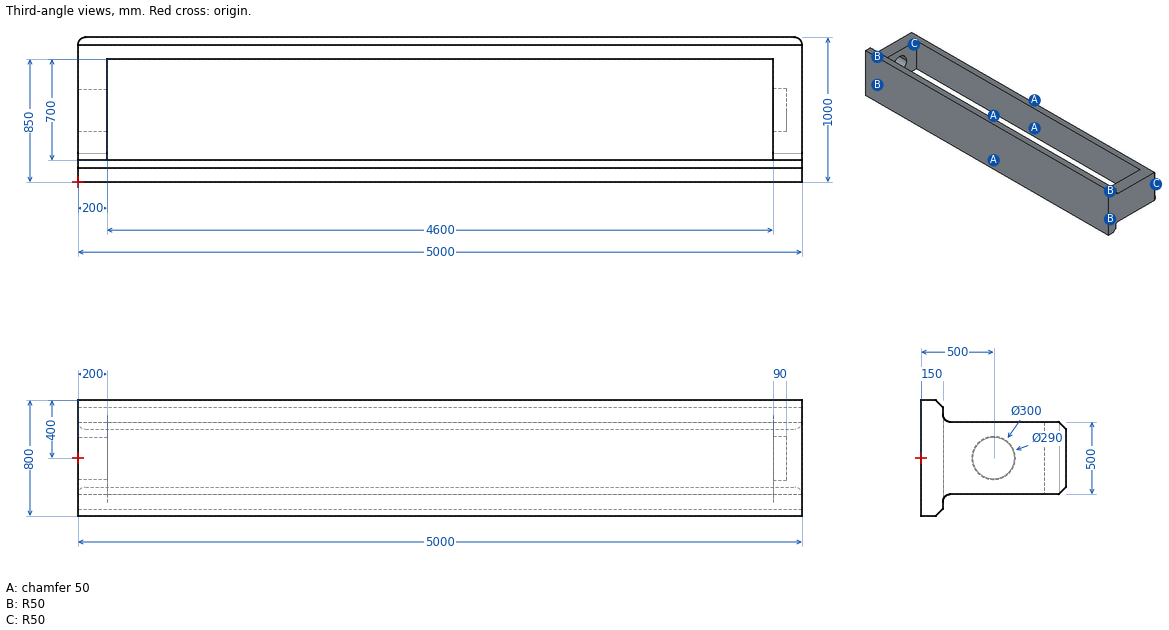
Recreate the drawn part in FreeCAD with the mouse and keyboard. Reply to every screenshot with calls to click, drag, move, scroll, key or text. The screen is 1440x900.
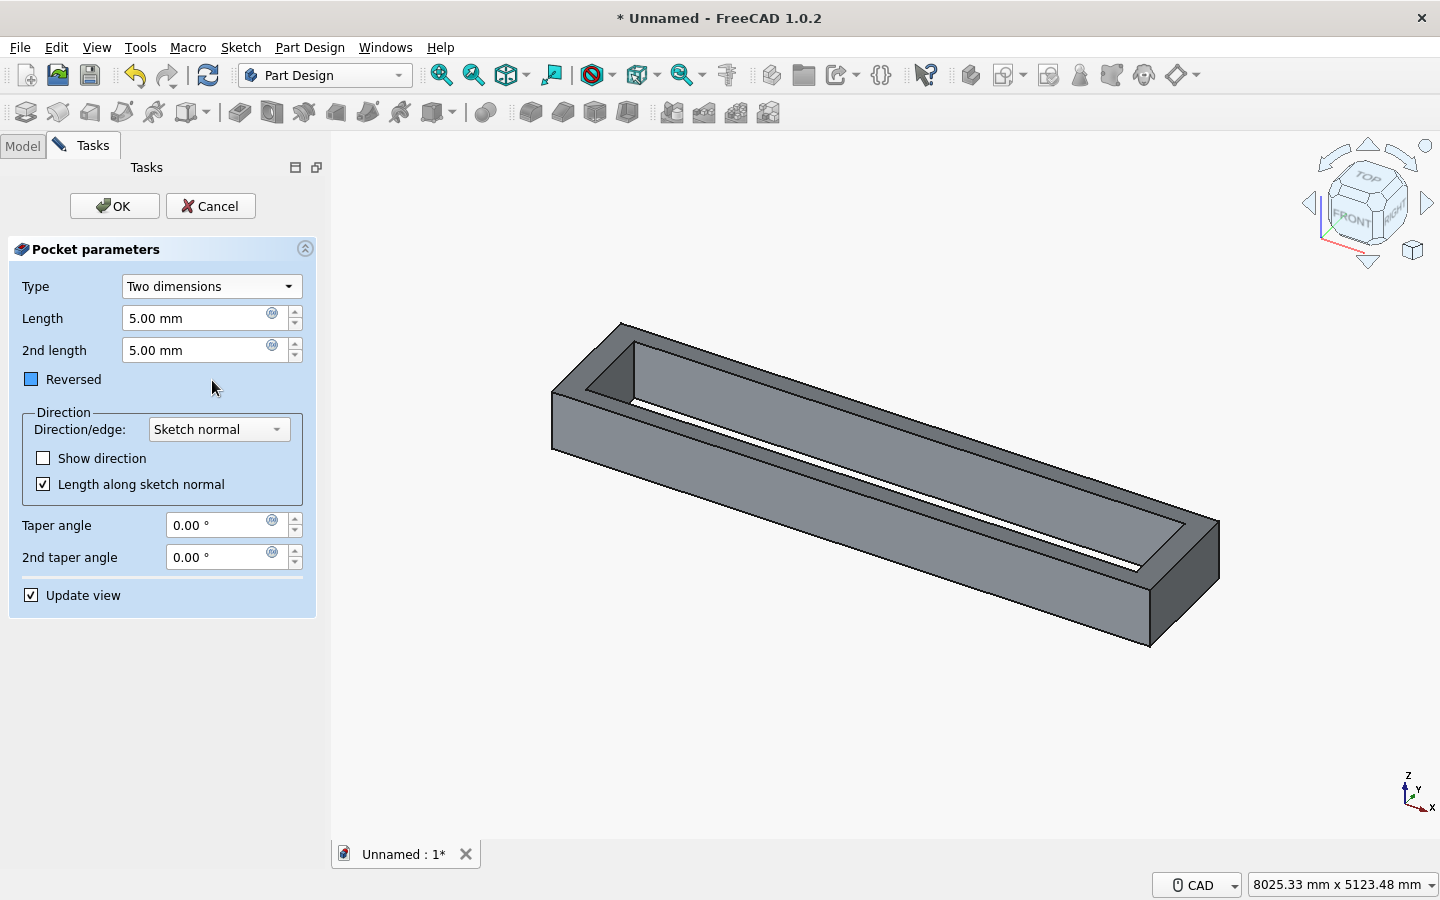
triple_click(204, 318)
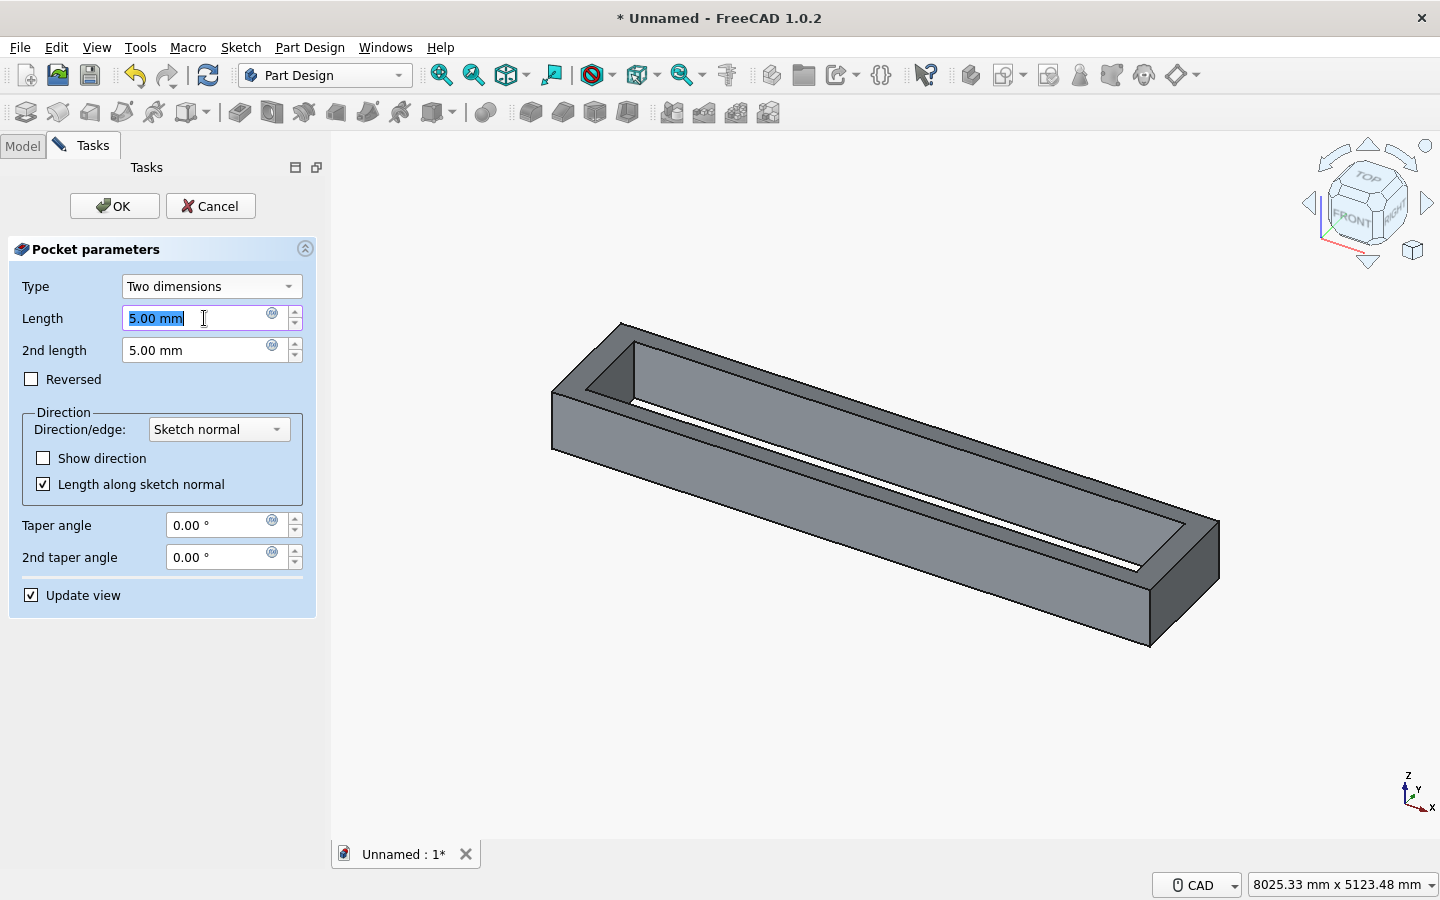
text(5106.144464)
key(Tab)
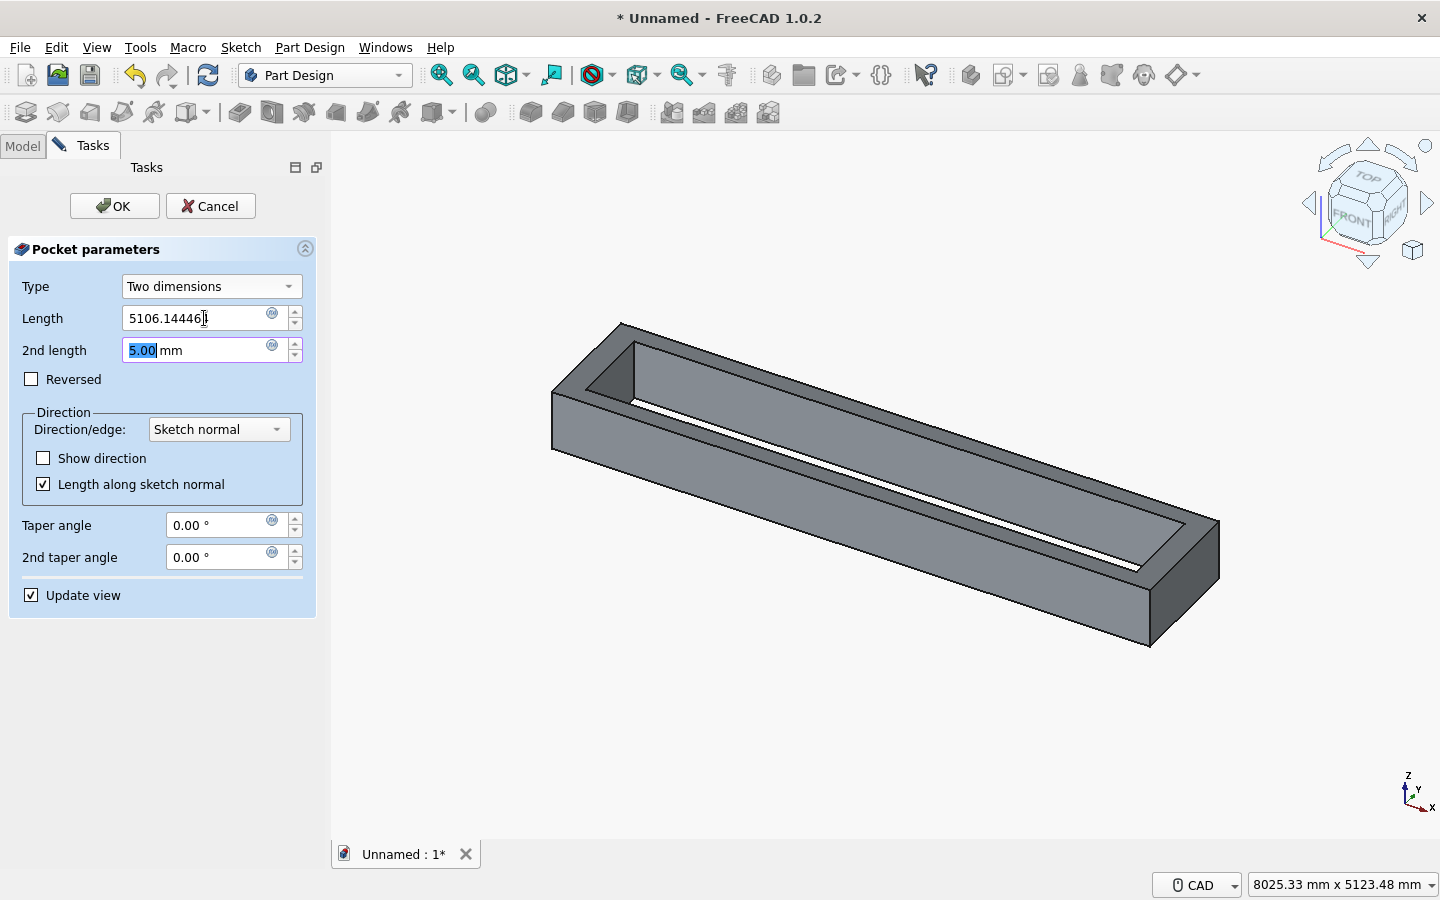
text(200)
key(Tab)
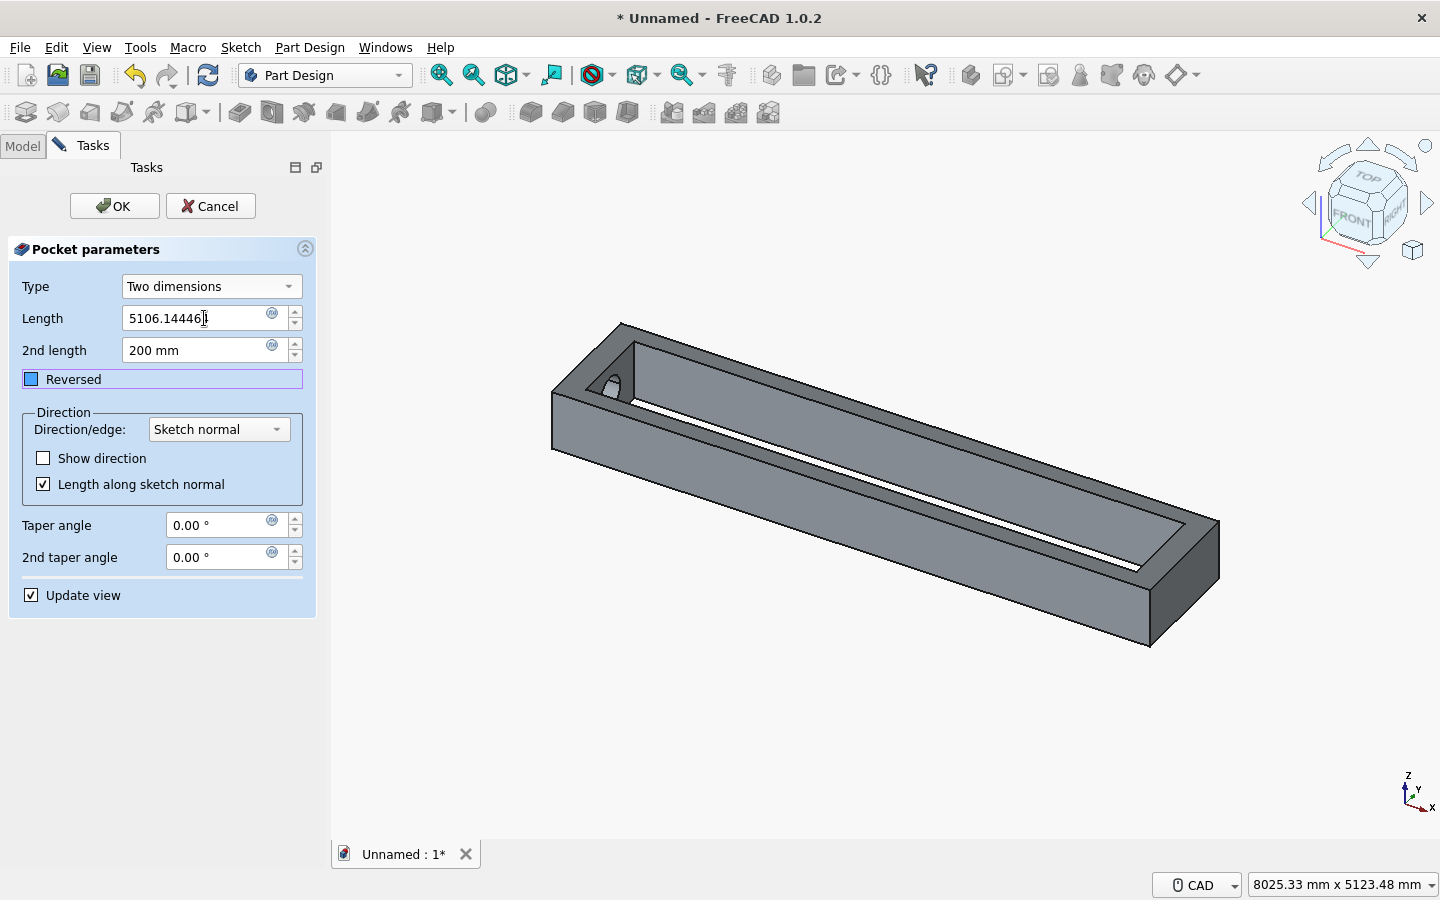
click(115, 206)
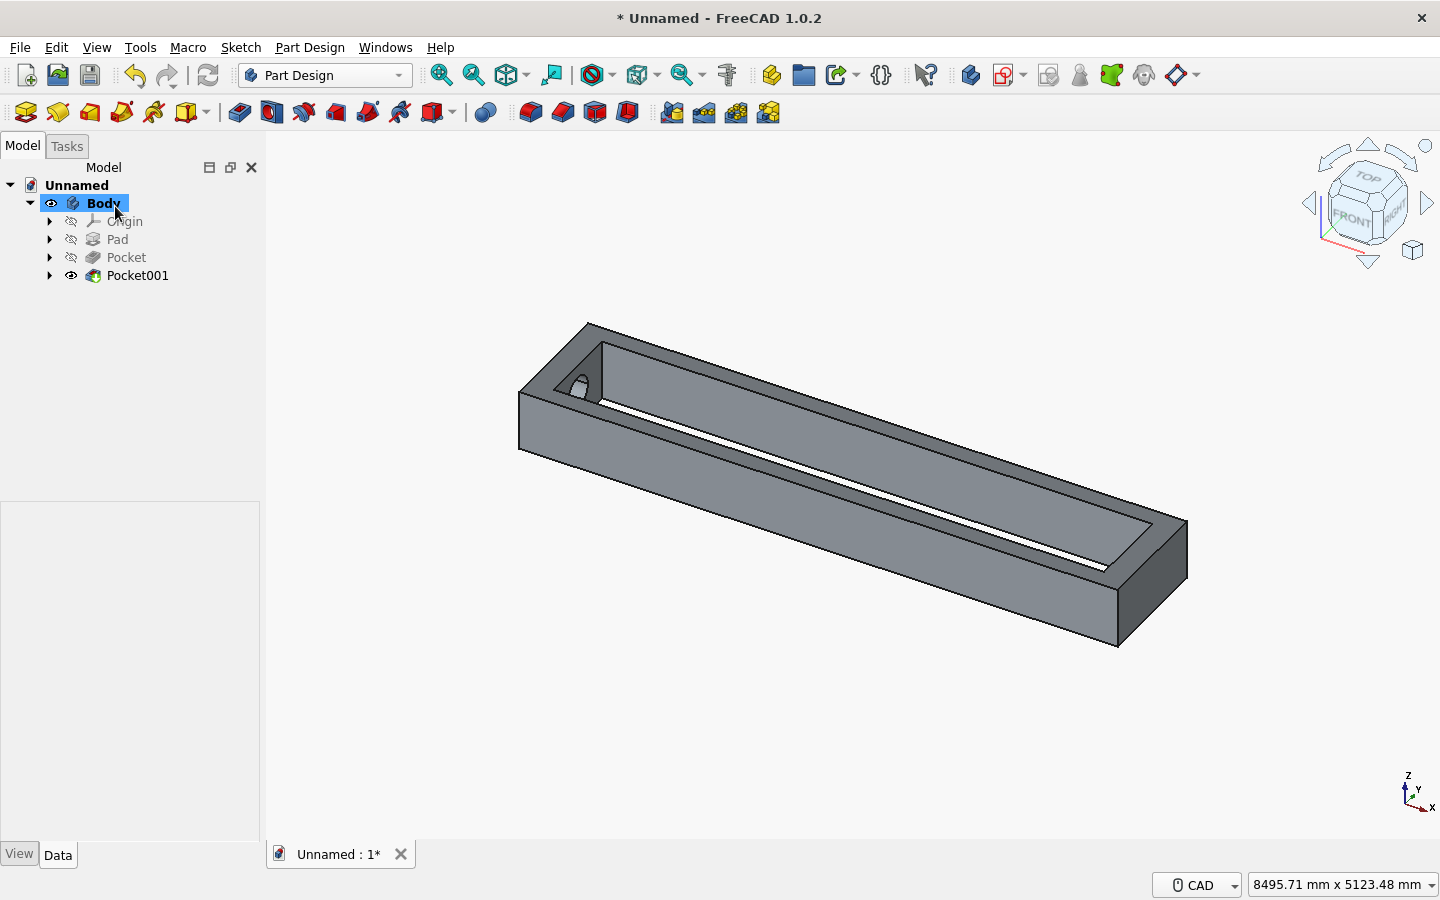
click(1075, 603)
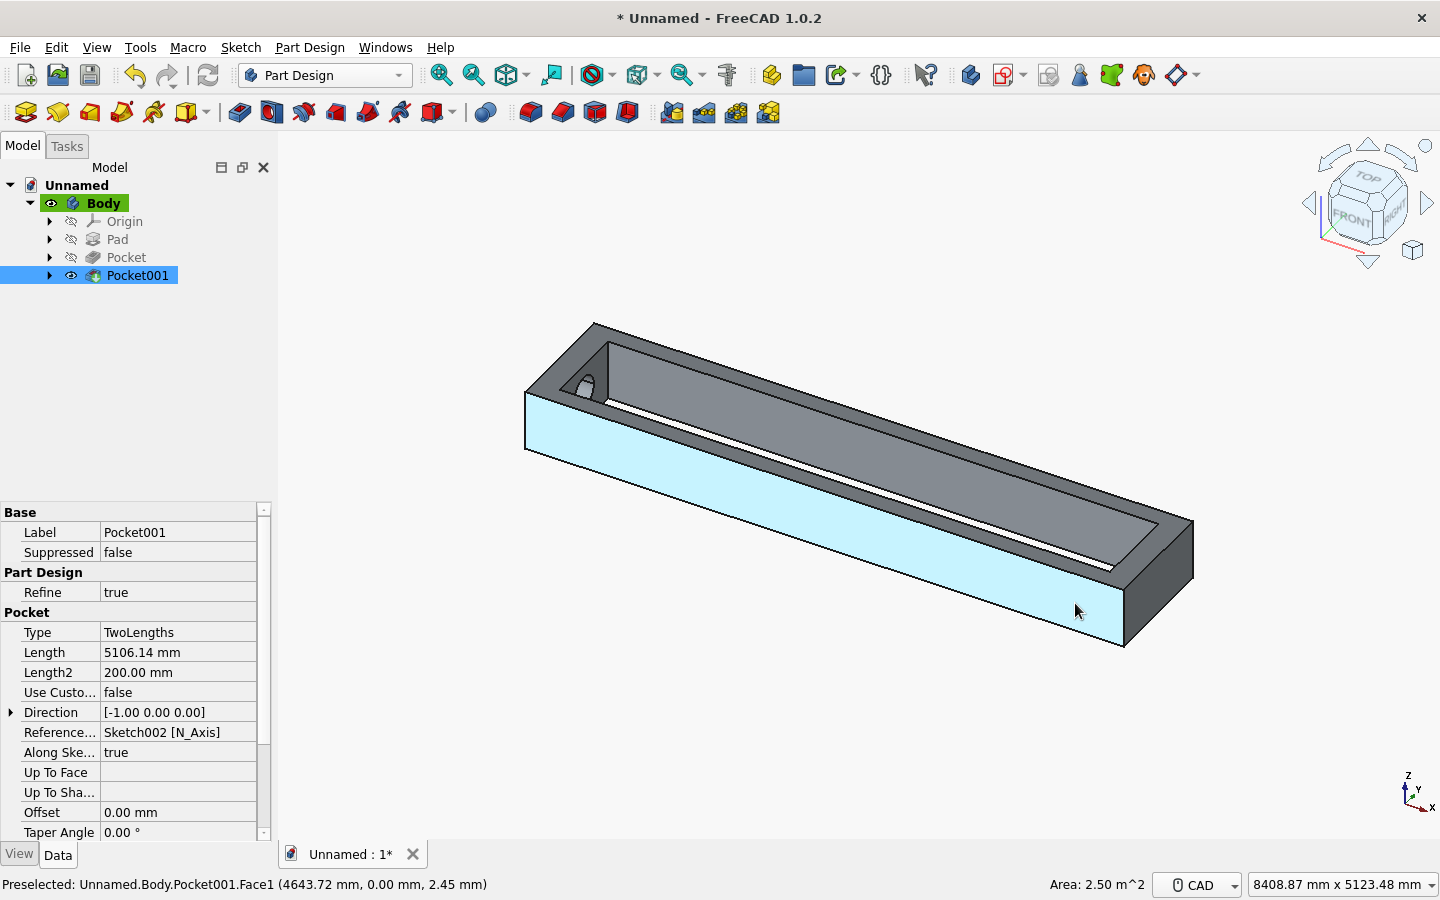
click(1004, 76)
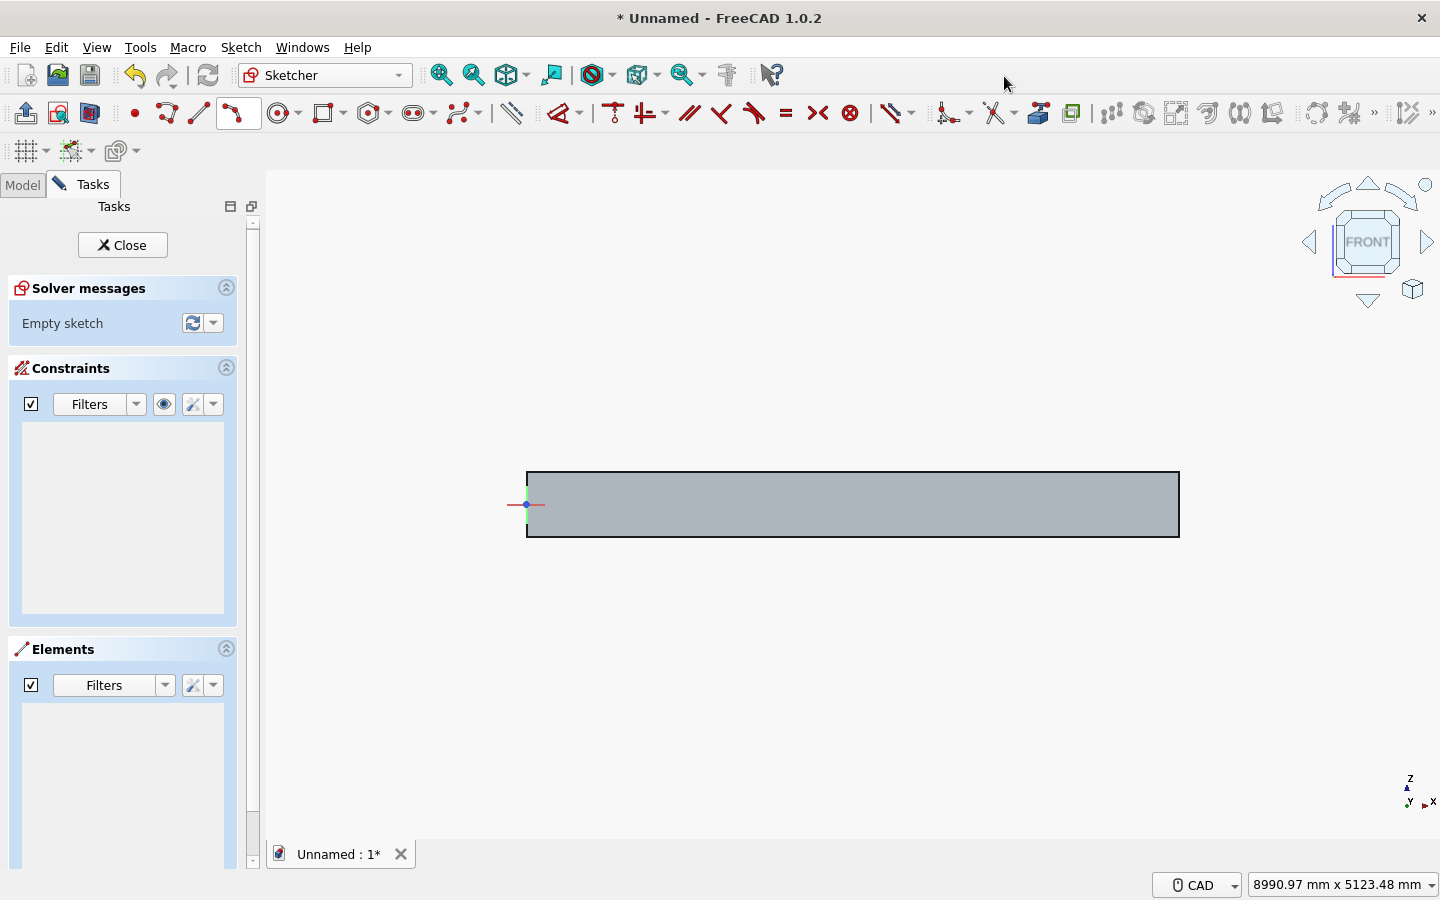
key(g)
key(r)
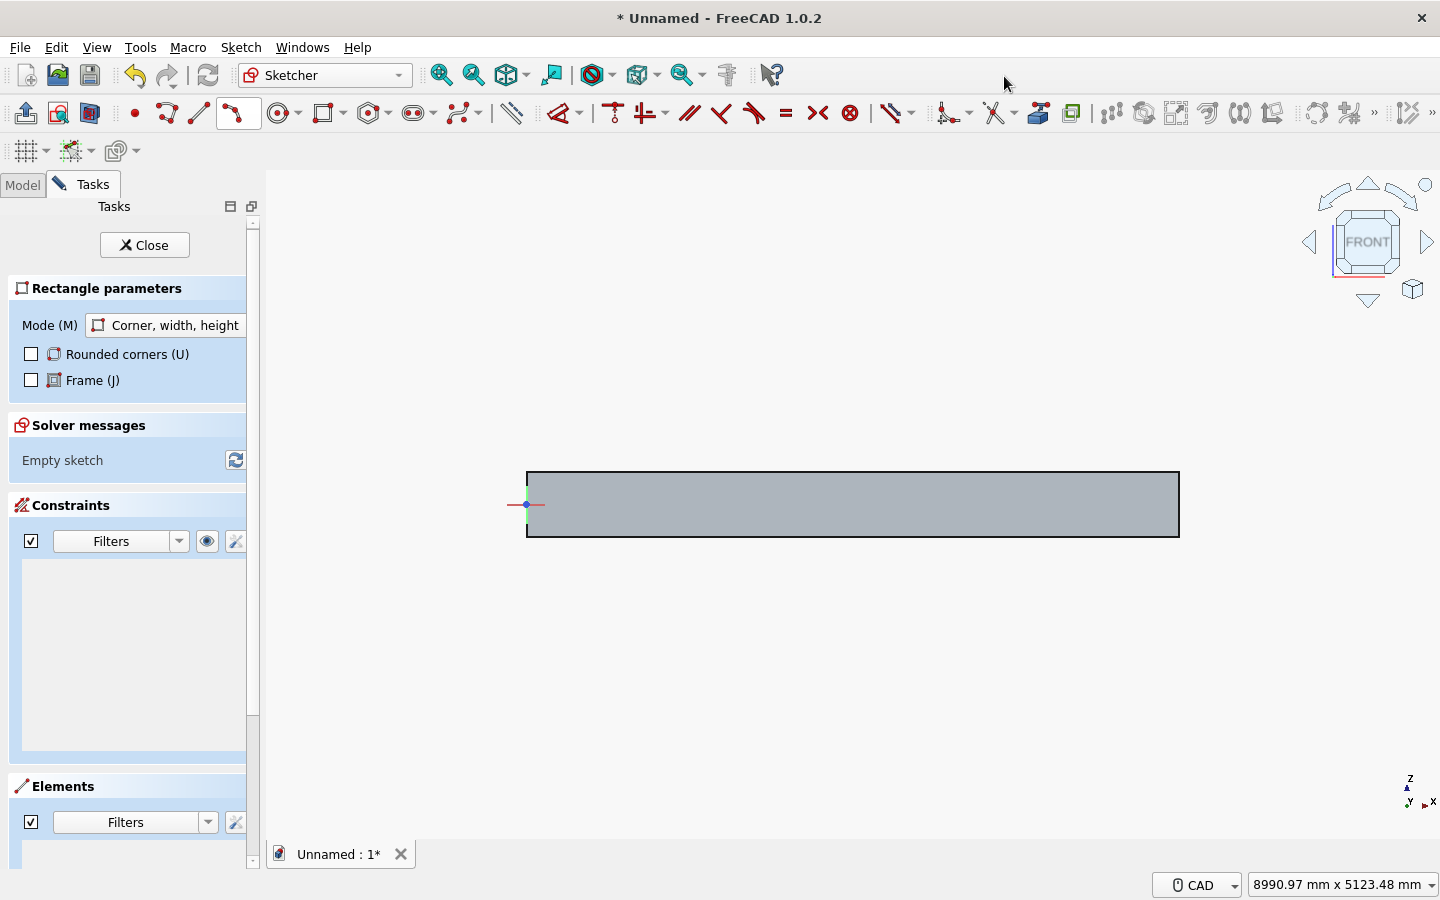
click(527, 452)
click(1179, 557)
key(Escape)